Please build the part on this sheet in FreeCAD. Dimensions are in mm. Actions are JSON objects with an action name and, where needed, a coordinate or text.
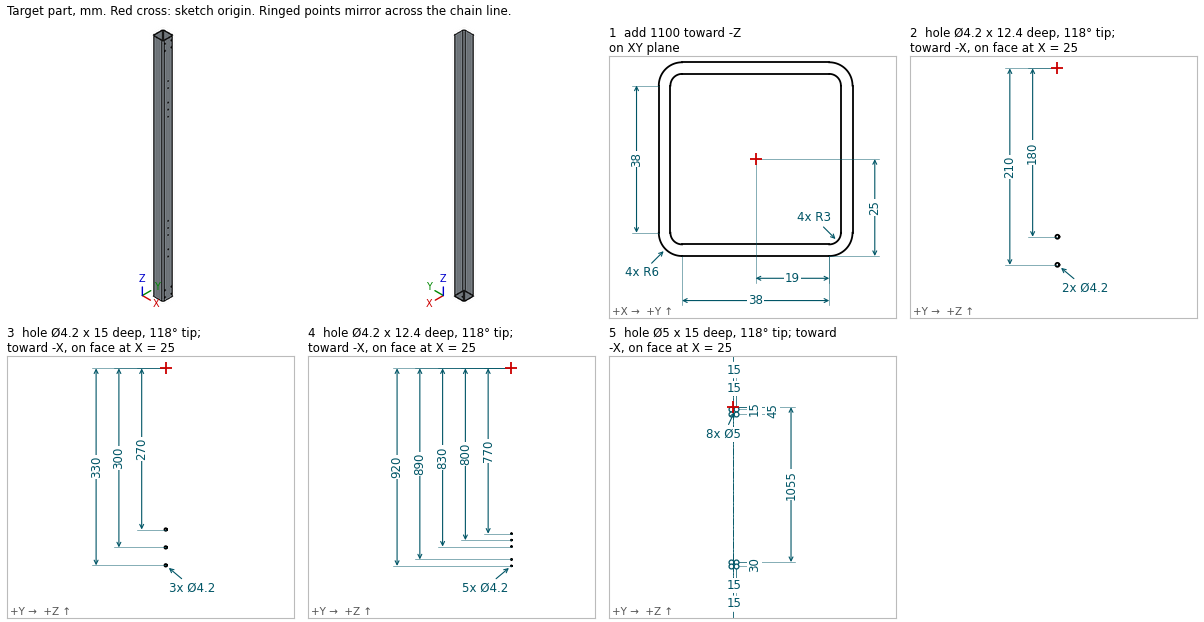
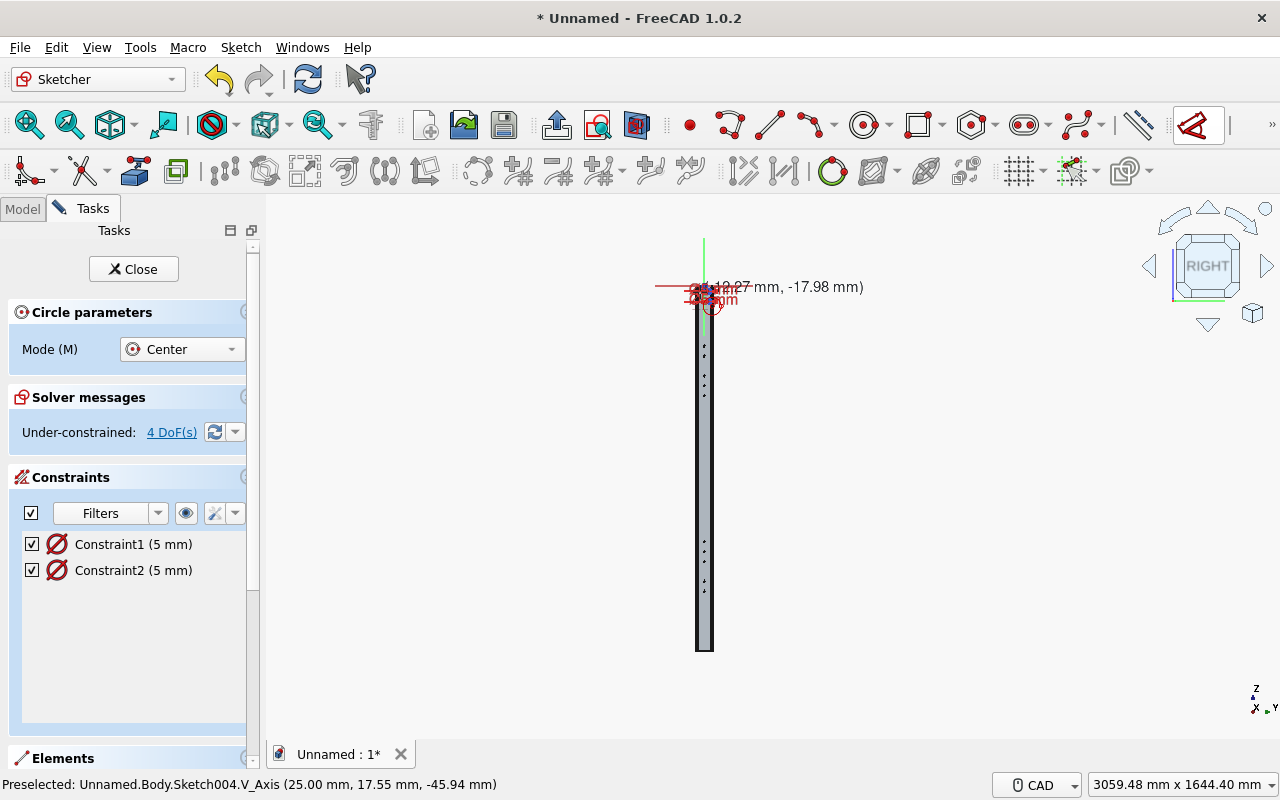
{"action": "scroll", "coordinate": [700, 291], "scroll_direction": "up", "scroll_amount": 6}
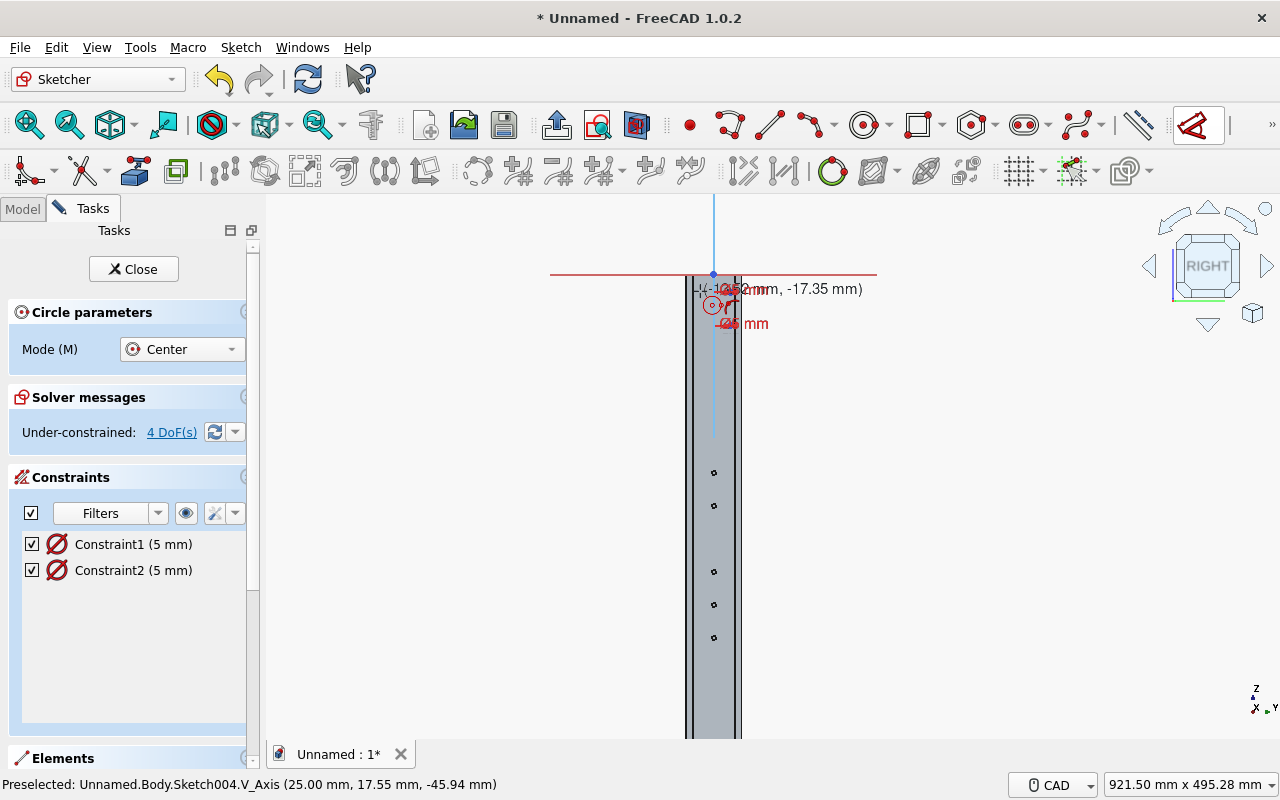
{"action": "left_click", "coordinate": [697, 291]}
{"action": "mouse_move", "coordinate": [699, 289]}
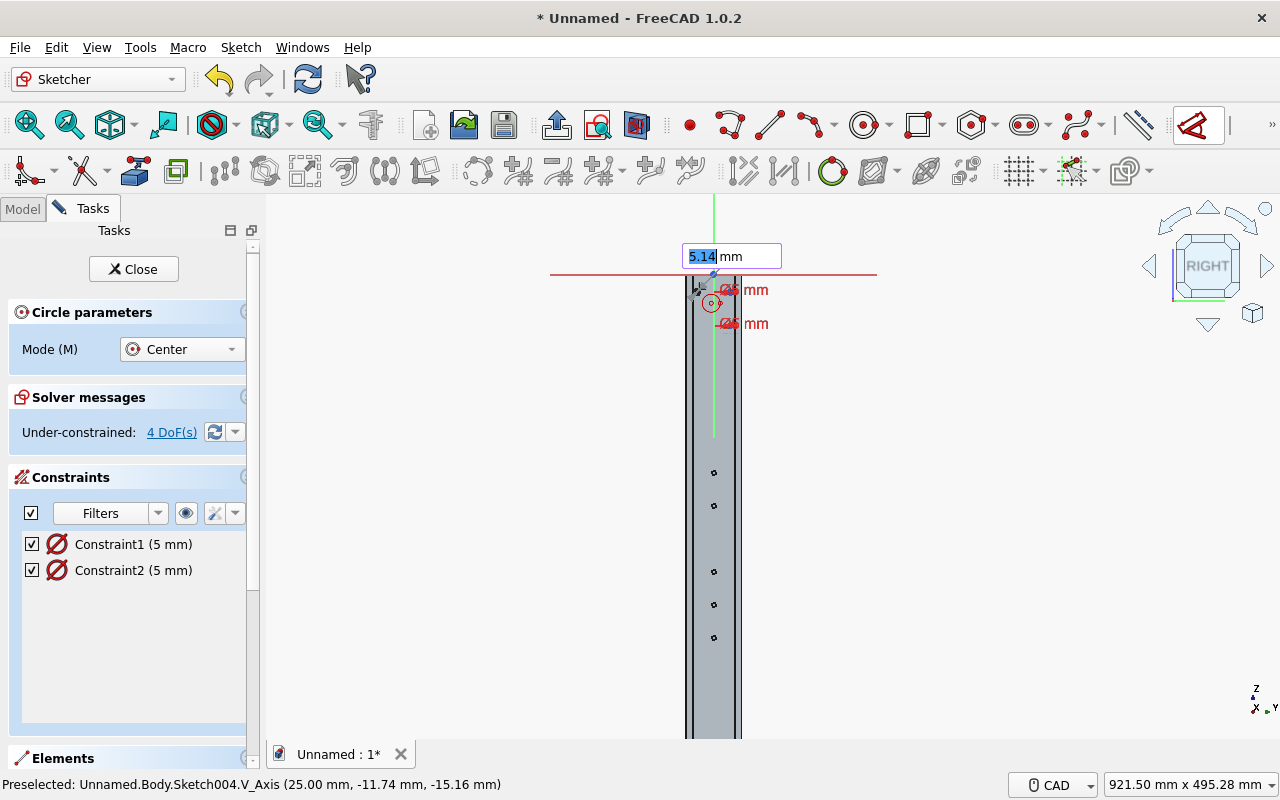
{"action": "type", "text": "5"}
{"action": "key", "text": "Return"}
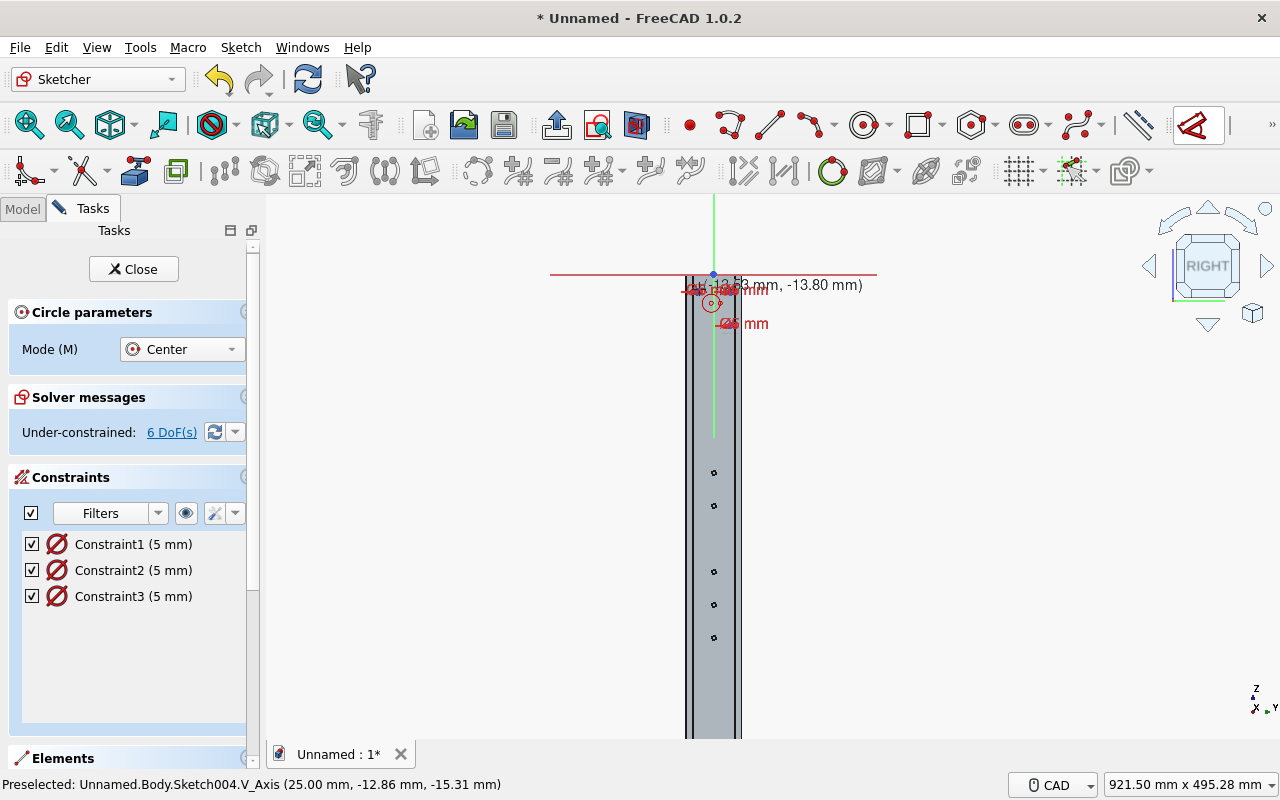
{"action": "scroll", "coordinate": [697, 324], "scroll_direction": "up", "scroll_amount": 11}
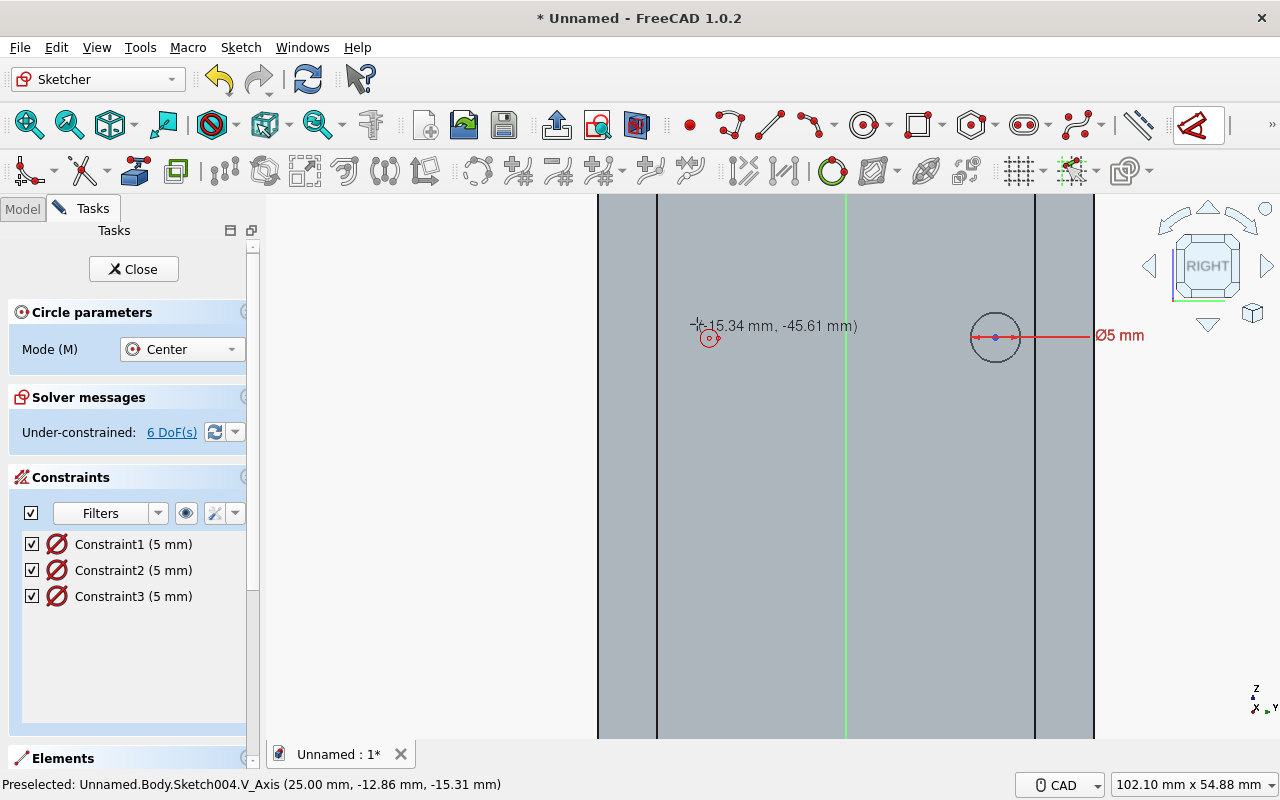
{"action": "scroll", "coordinate": [700, 300], "scroll_direction": "down", "scroll_amount": 17}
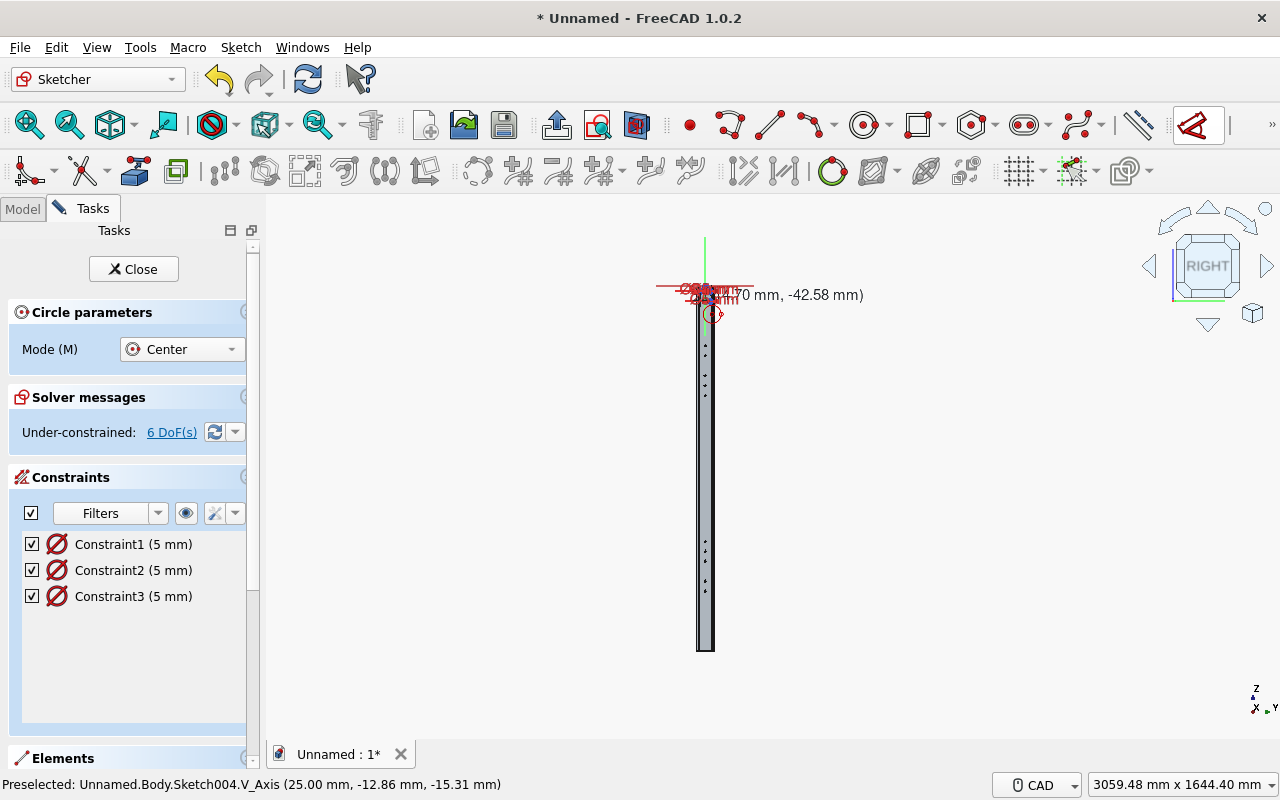
{"action": "scroll", "coordinate": [700, 301], "scroll_direction": "up", "scroll_amount": 6}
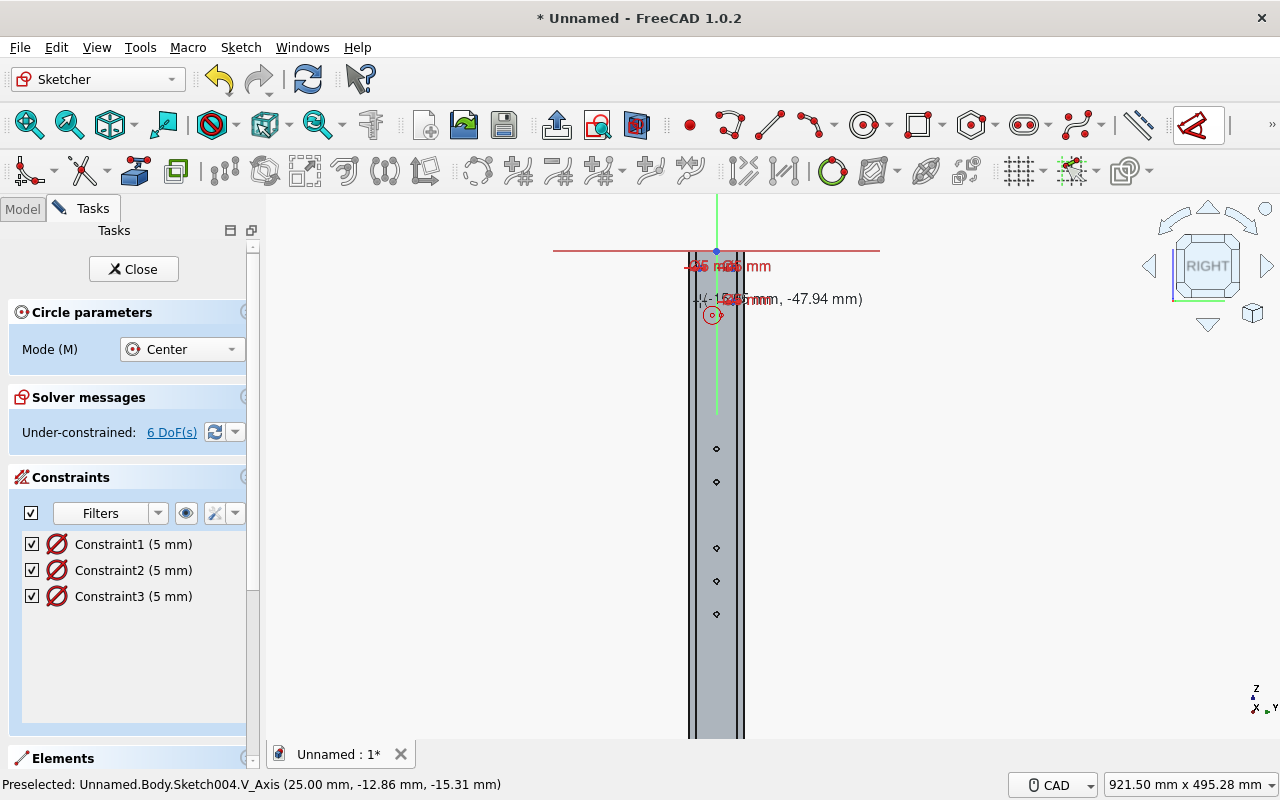
{"action": "left_click", "coordinate": [700, 301]}
{"action": "mouse_move", "coordinate": [702, 299]}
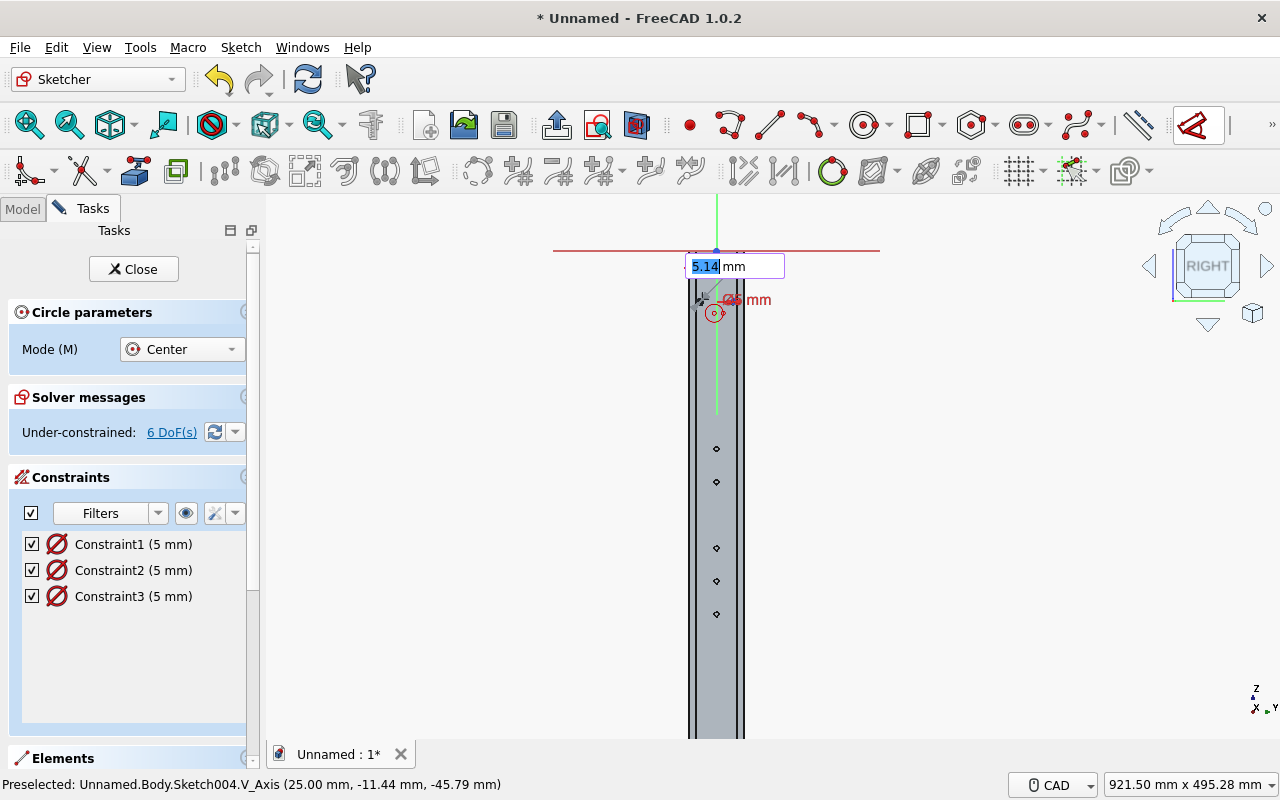
{"action": "type", "text": "5"}
{"action": "key", "text": "Return"}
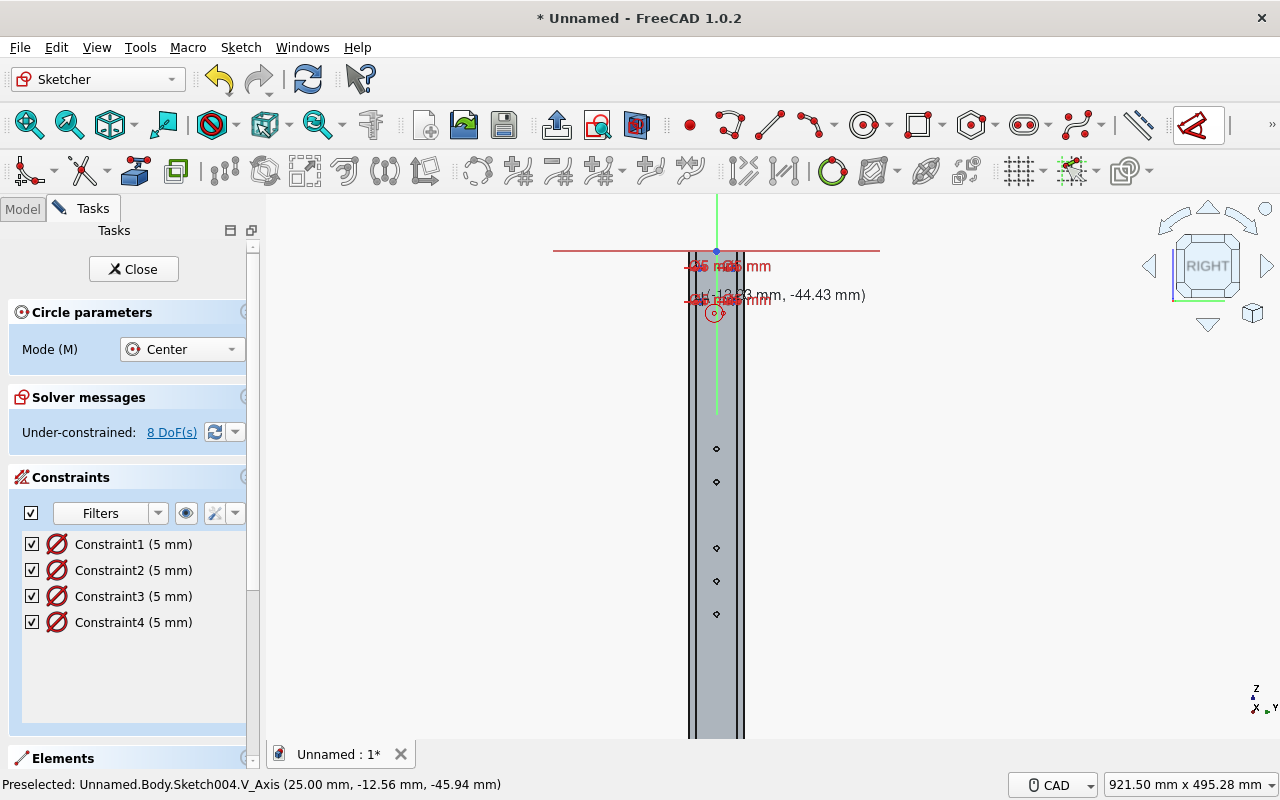
{"action": "scroll", "coordinate": [699, 301], "scroll_direction": "down", "scroll_amount": 6}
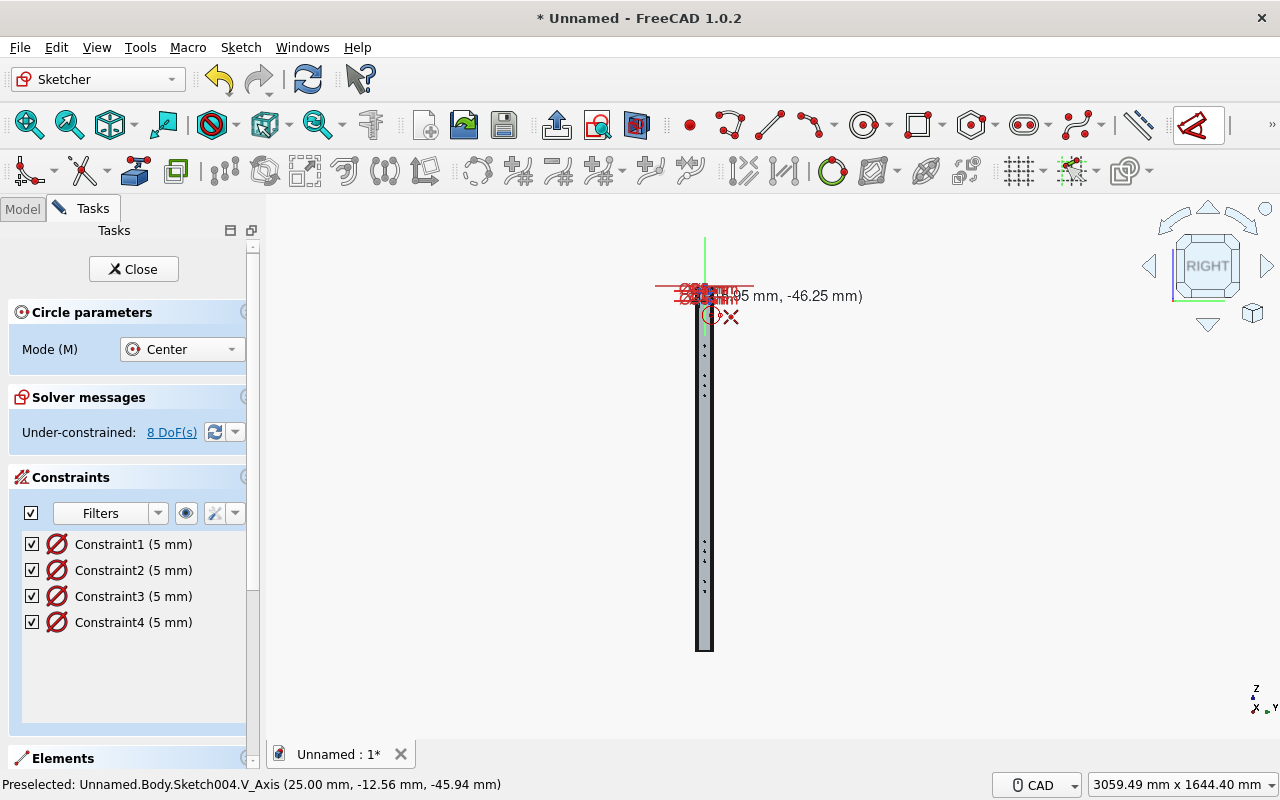
{"action": "scroll", "coordinate": [710, 636], "scroll_direction": "up", "scroll_amount": 17}